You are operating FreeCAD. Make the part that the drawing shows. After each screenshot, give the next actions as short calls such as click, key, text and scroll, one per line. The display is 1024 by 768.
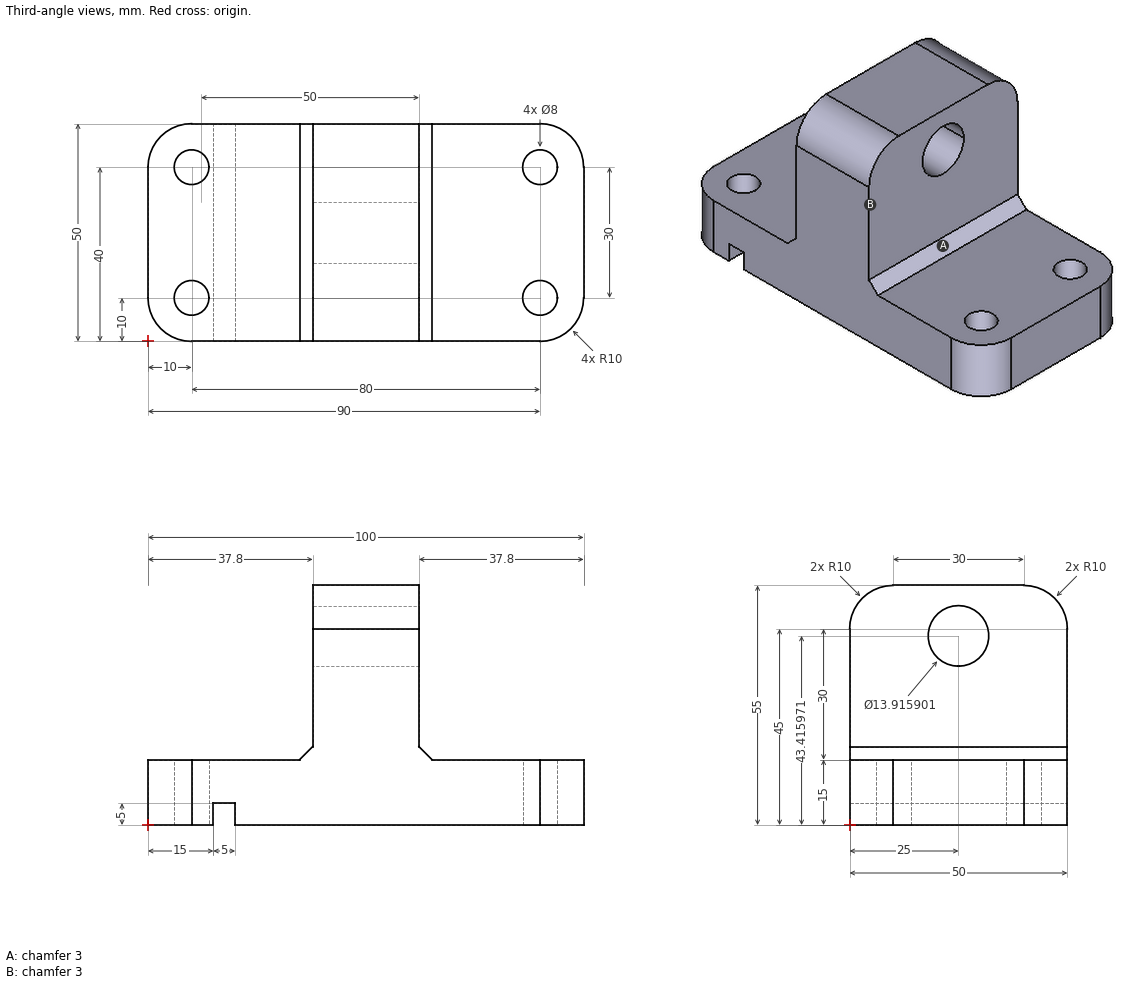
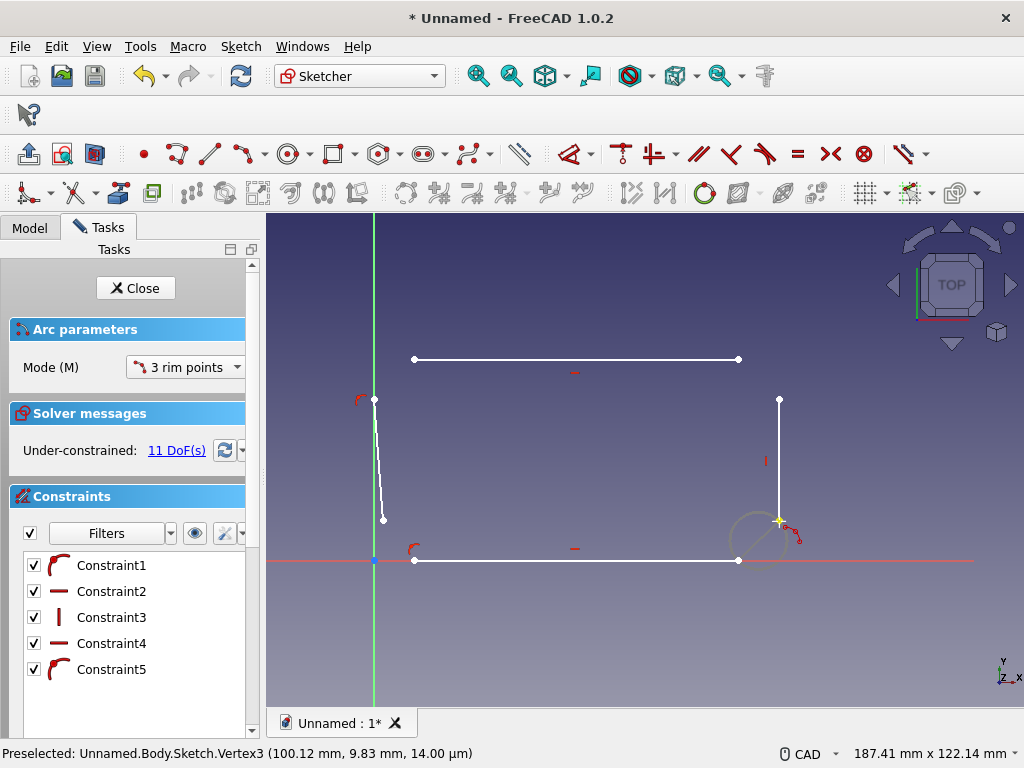
scroll(767, 549, up, 2)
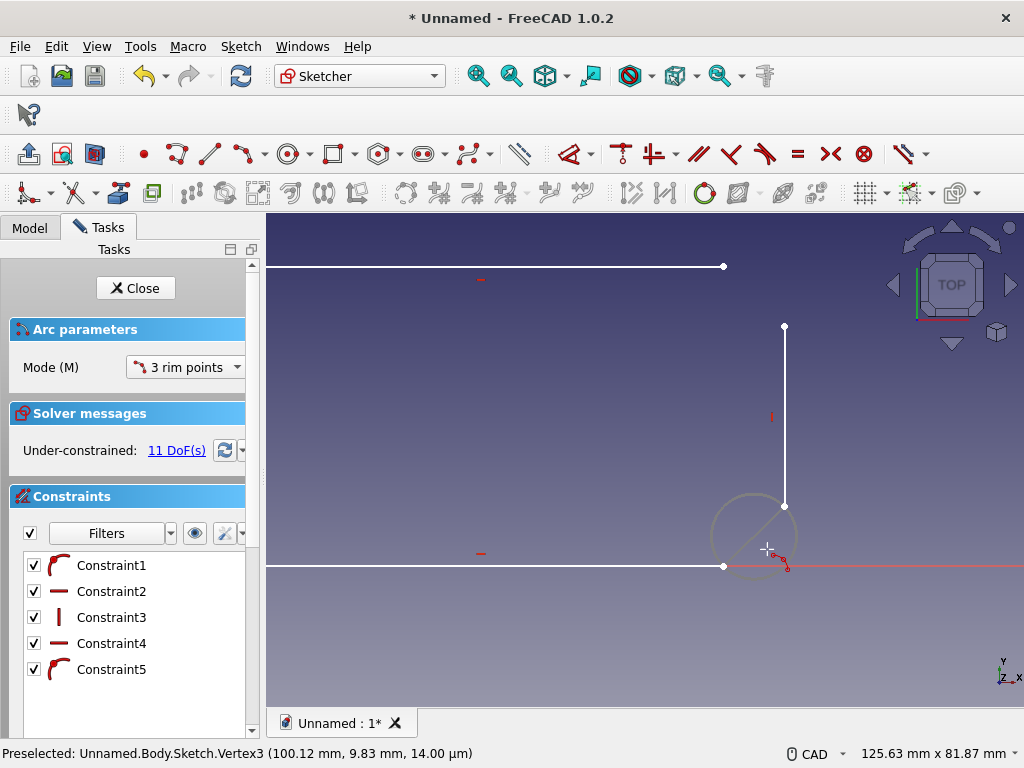
click(766, 549)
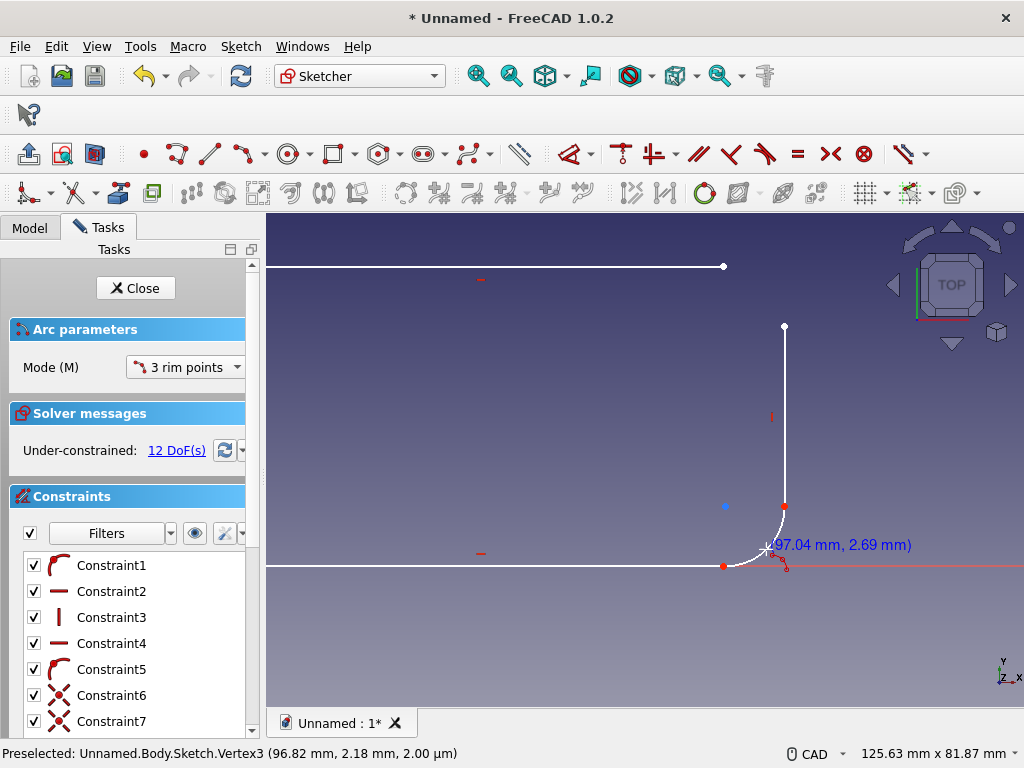
click(785, 326)
click(723, 267)
click(766, 282)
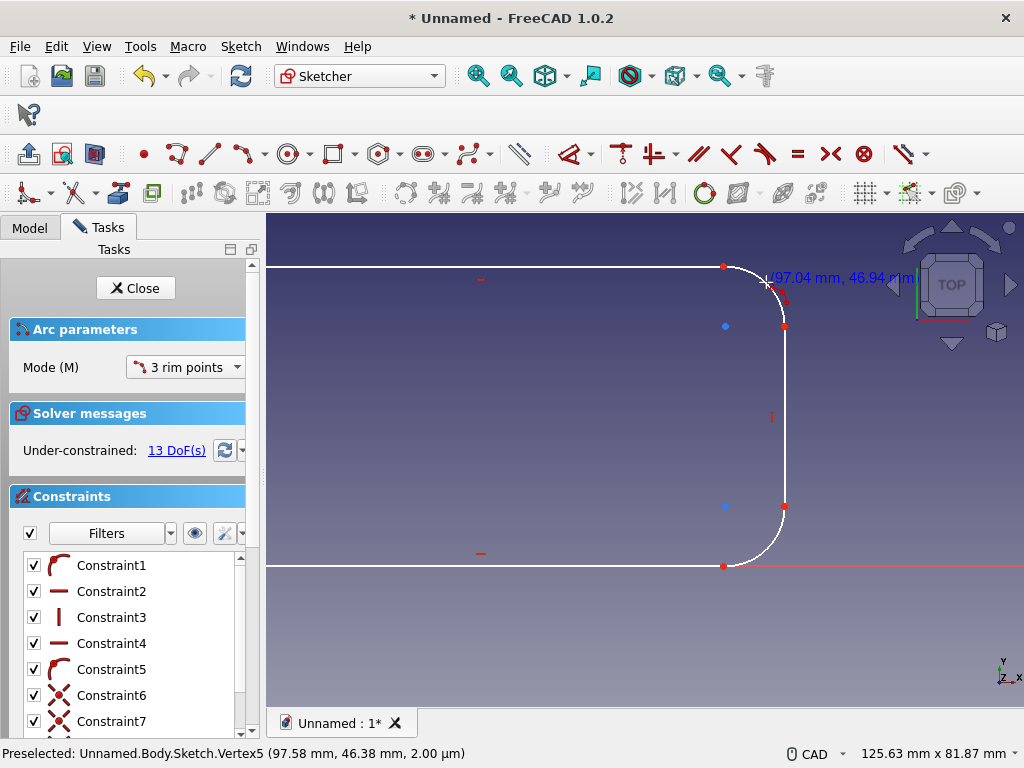
scroll(768, 551, down, 2)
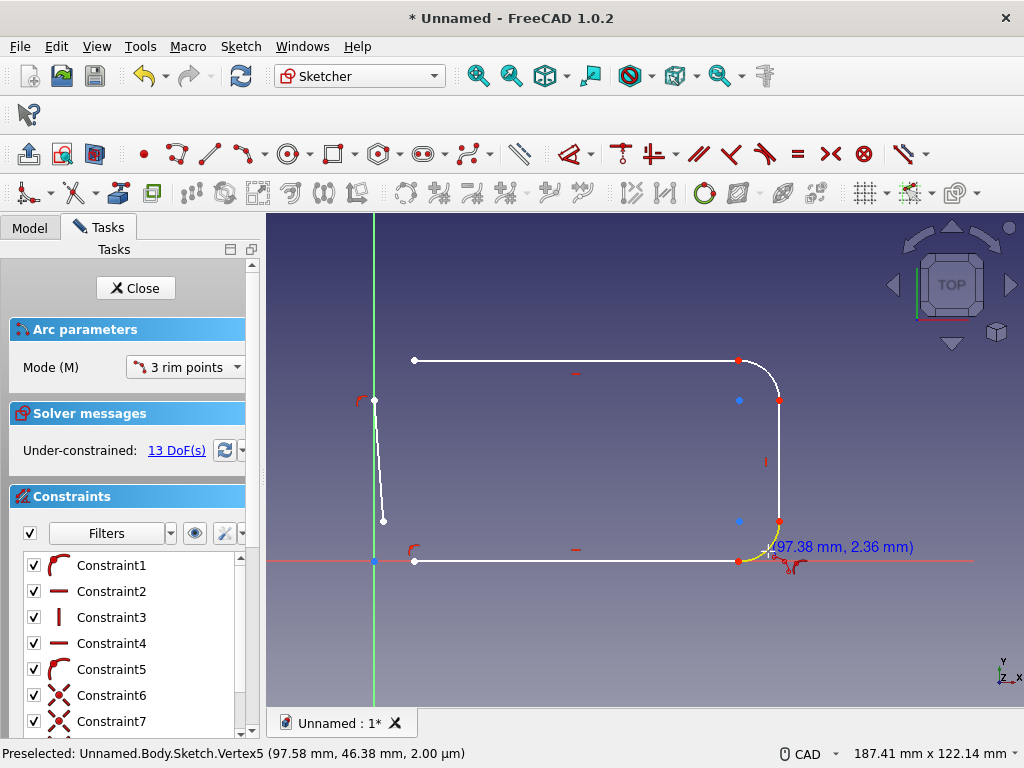
click(414, 361)
click(374, 401)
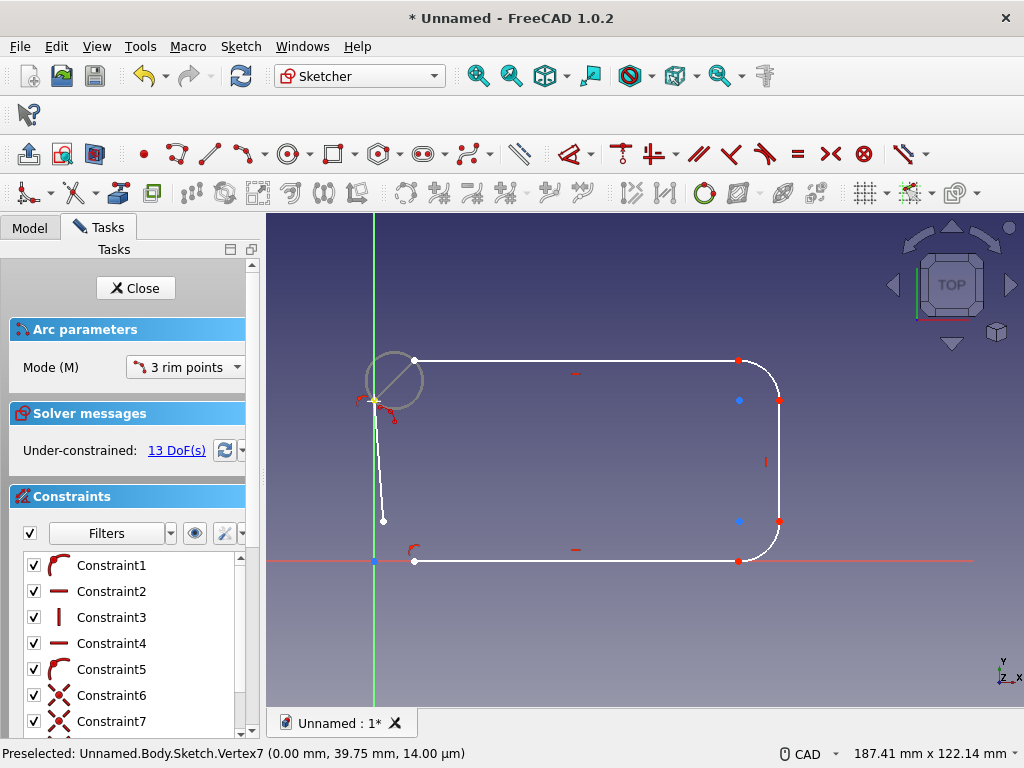
scroll(386, 371, up, 2)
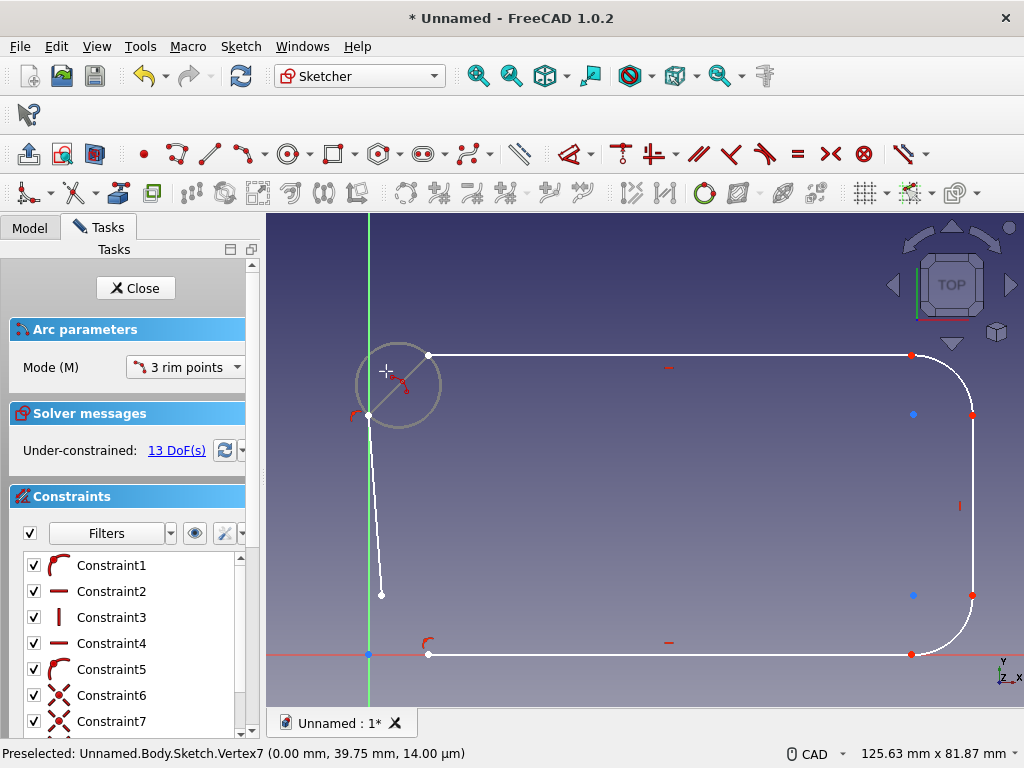
click(386, 371)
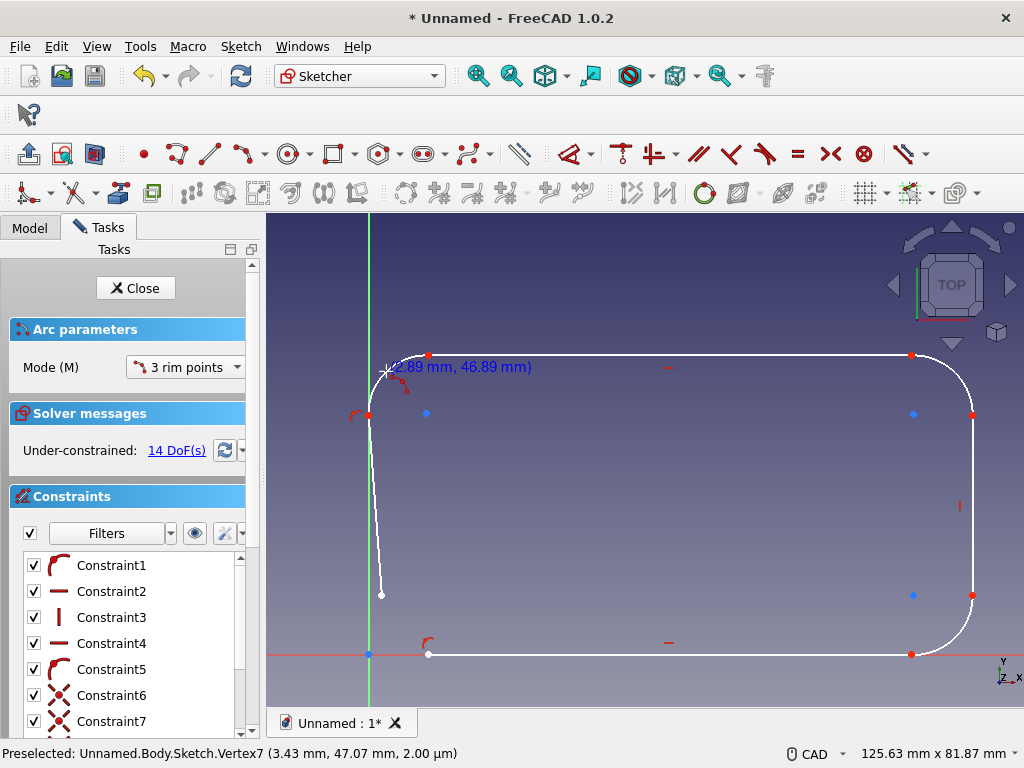
click(382, 596)
click(428, 655)
click(386, 637)
key(Escape)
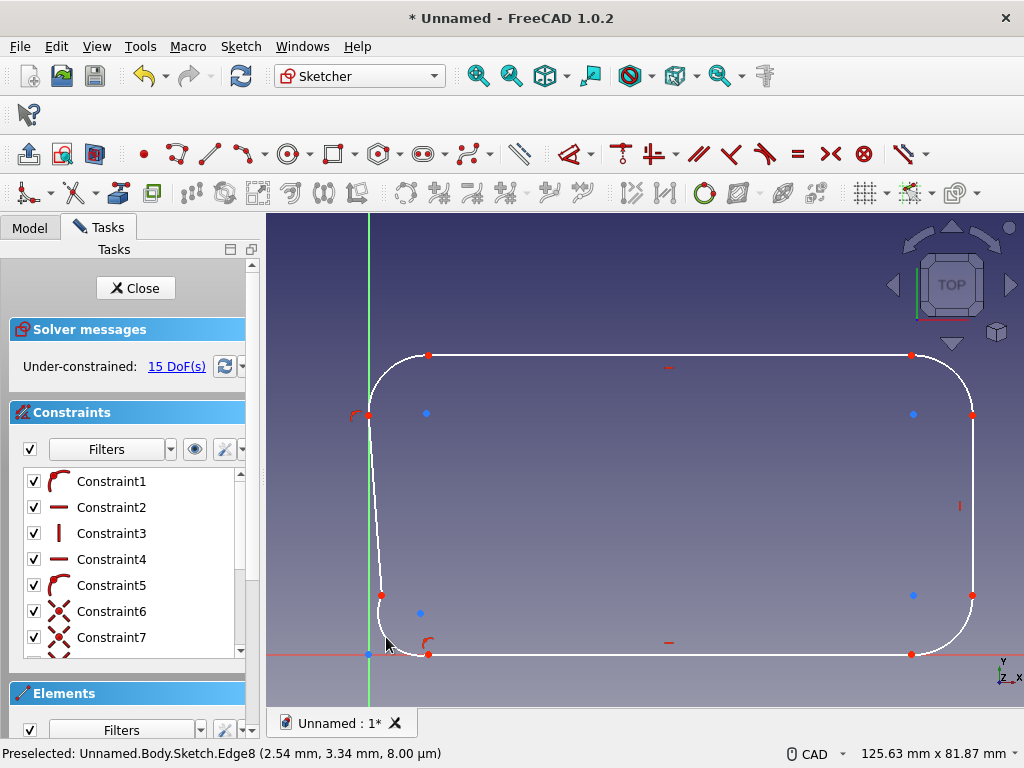
click(573, 655)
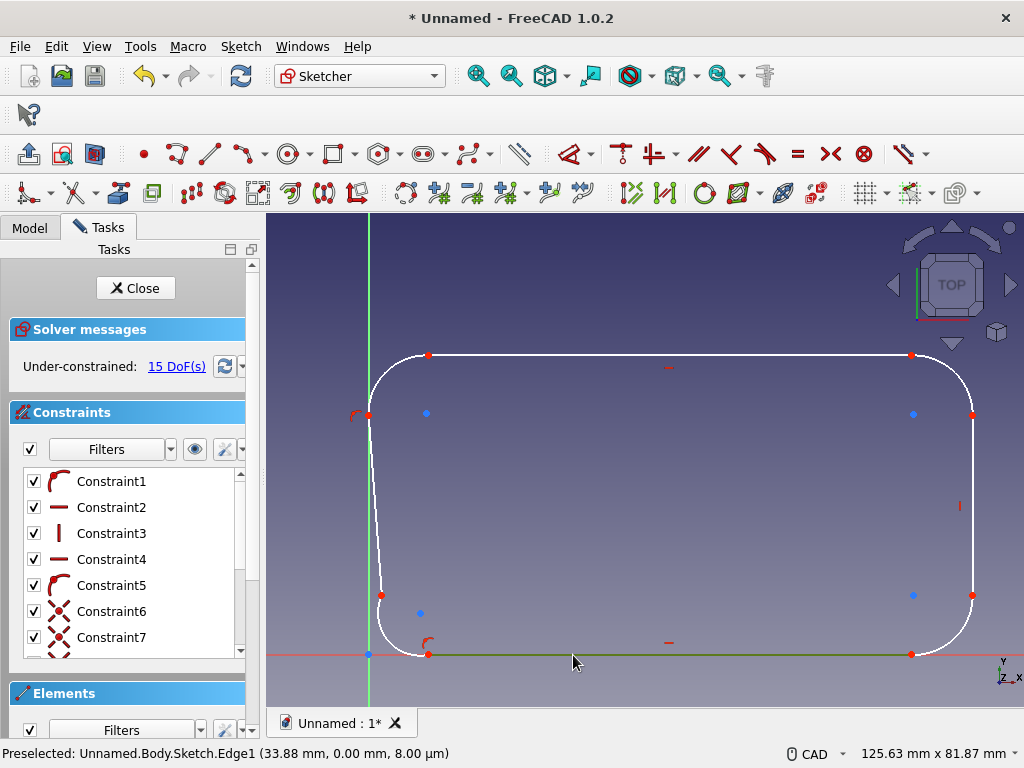
scroll(386, 370, down, 2)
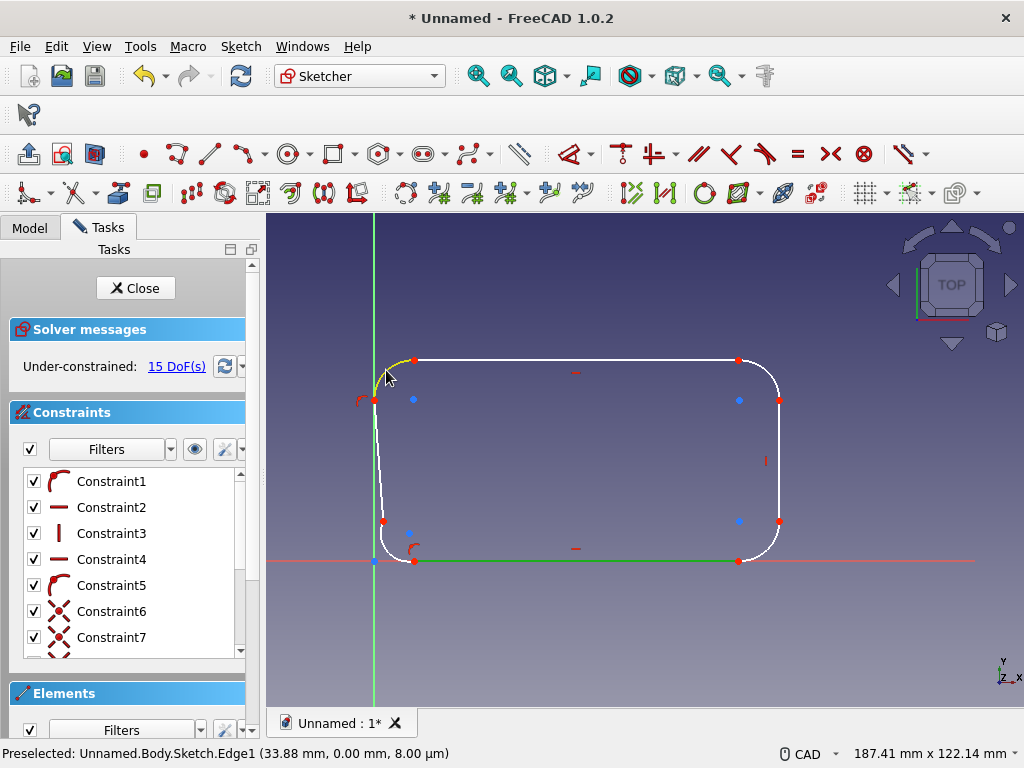
click(775, 540)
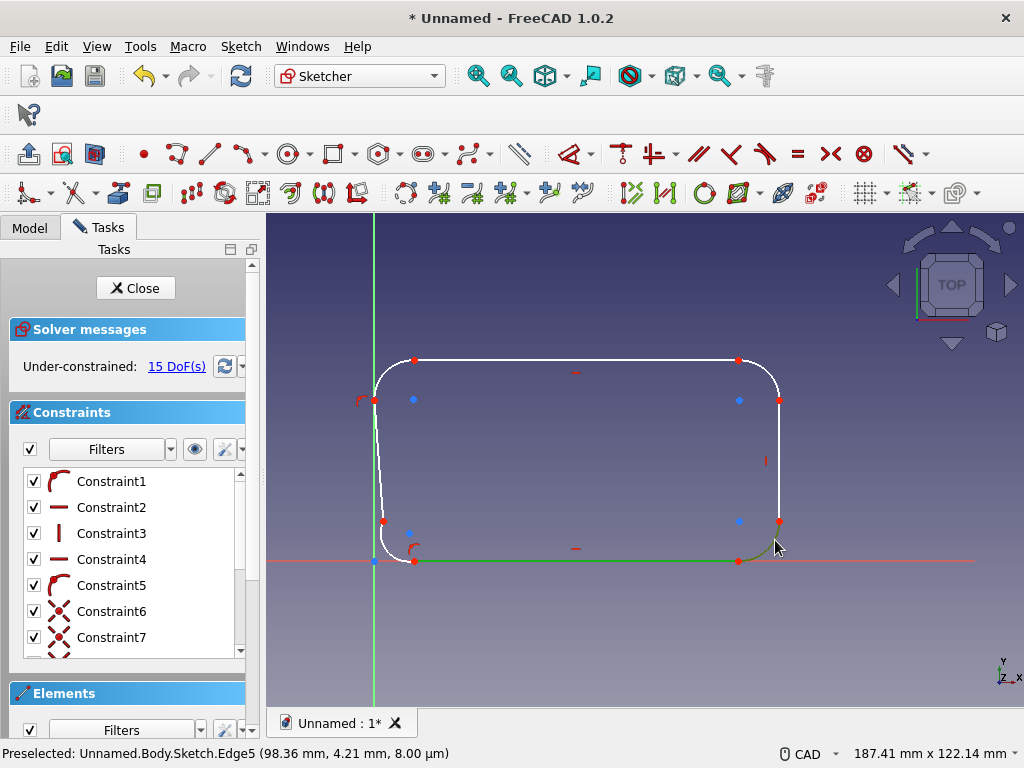
click(765, 154)